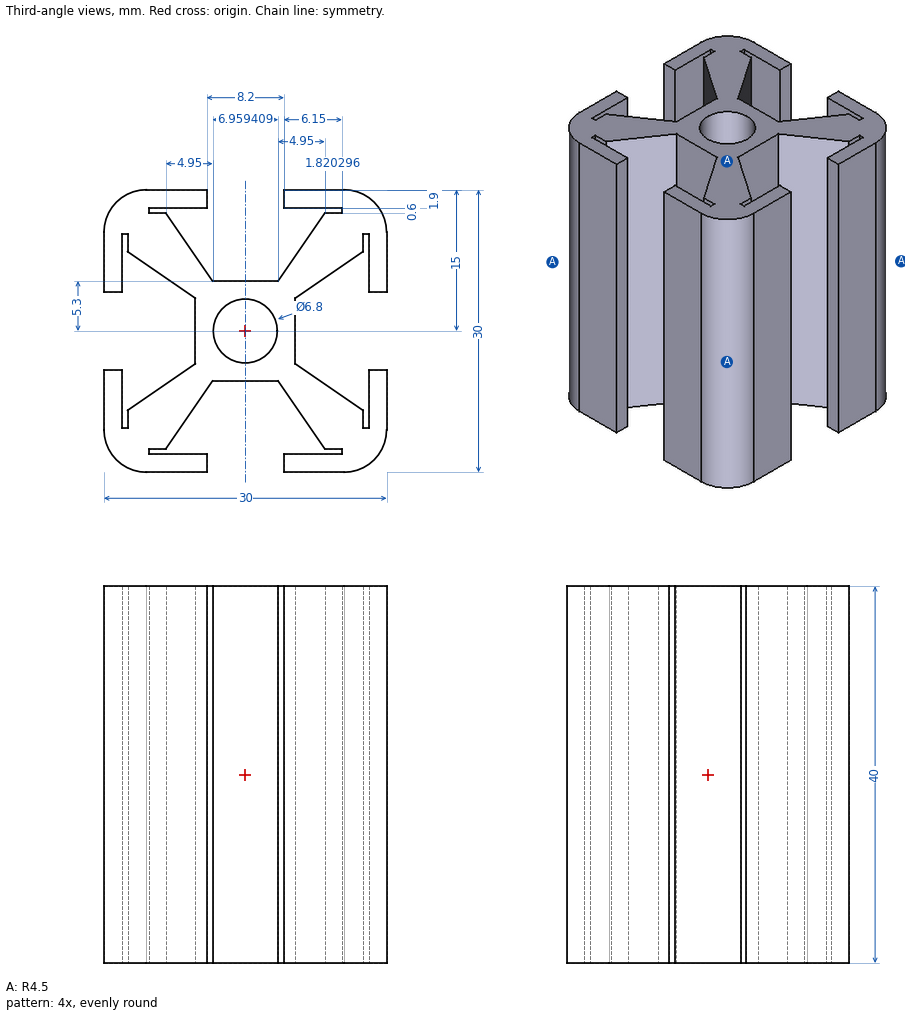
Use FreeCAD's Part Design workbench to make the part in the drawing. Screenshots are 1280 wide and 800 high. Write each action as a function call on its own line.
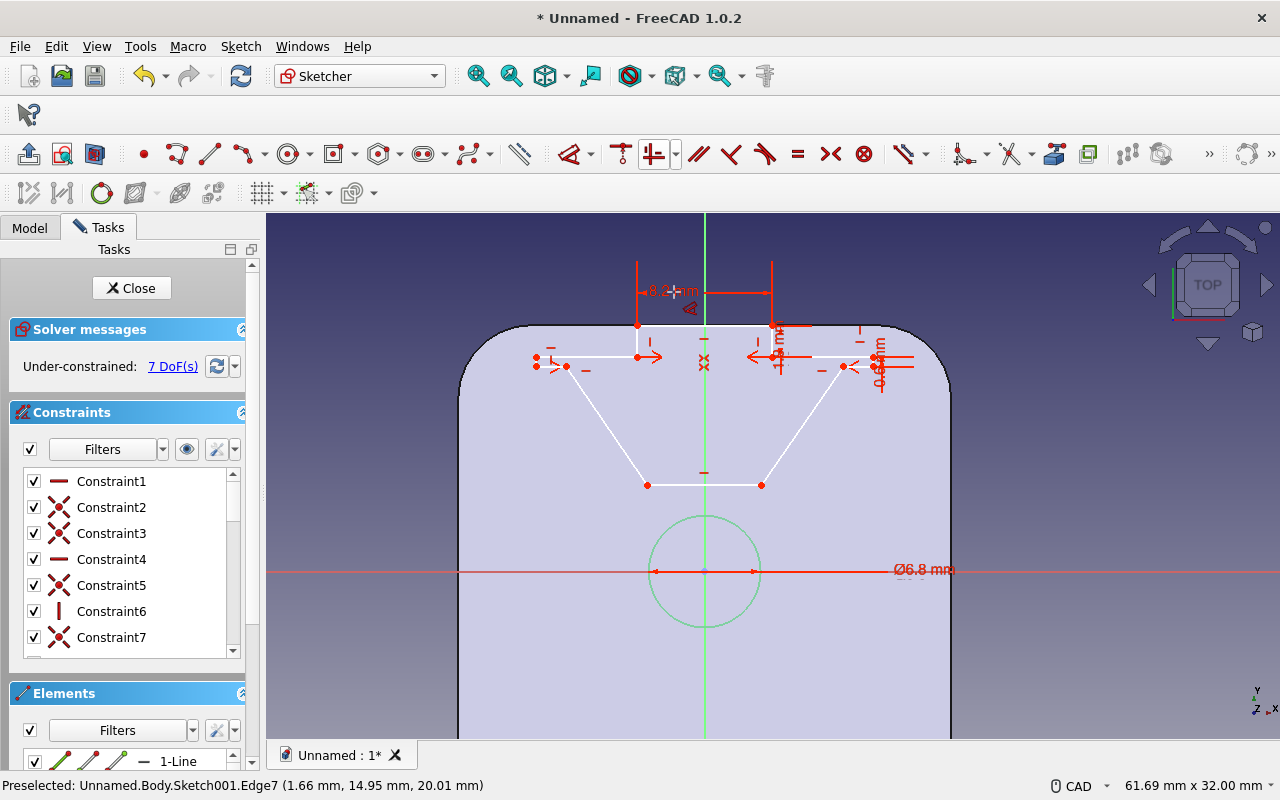
click(772, 326)
click(806, 449)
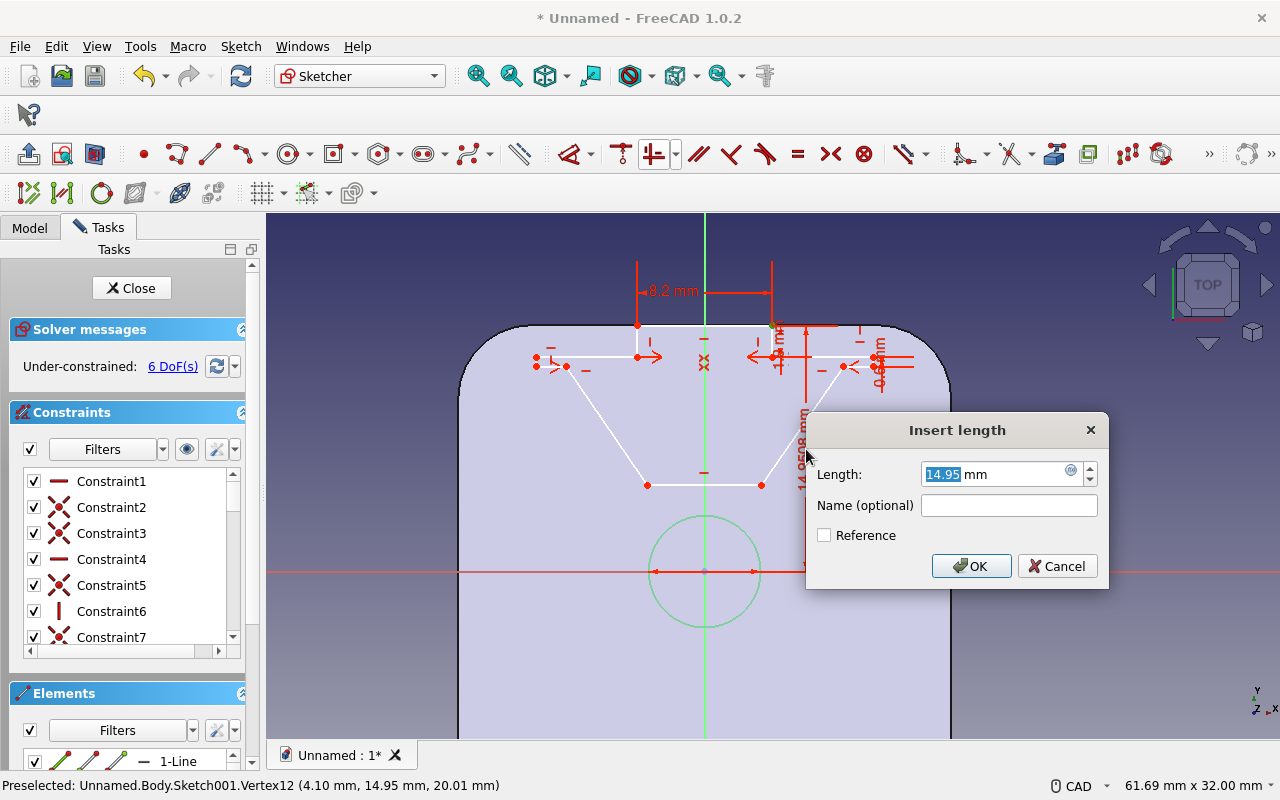
text(15)
key(Return)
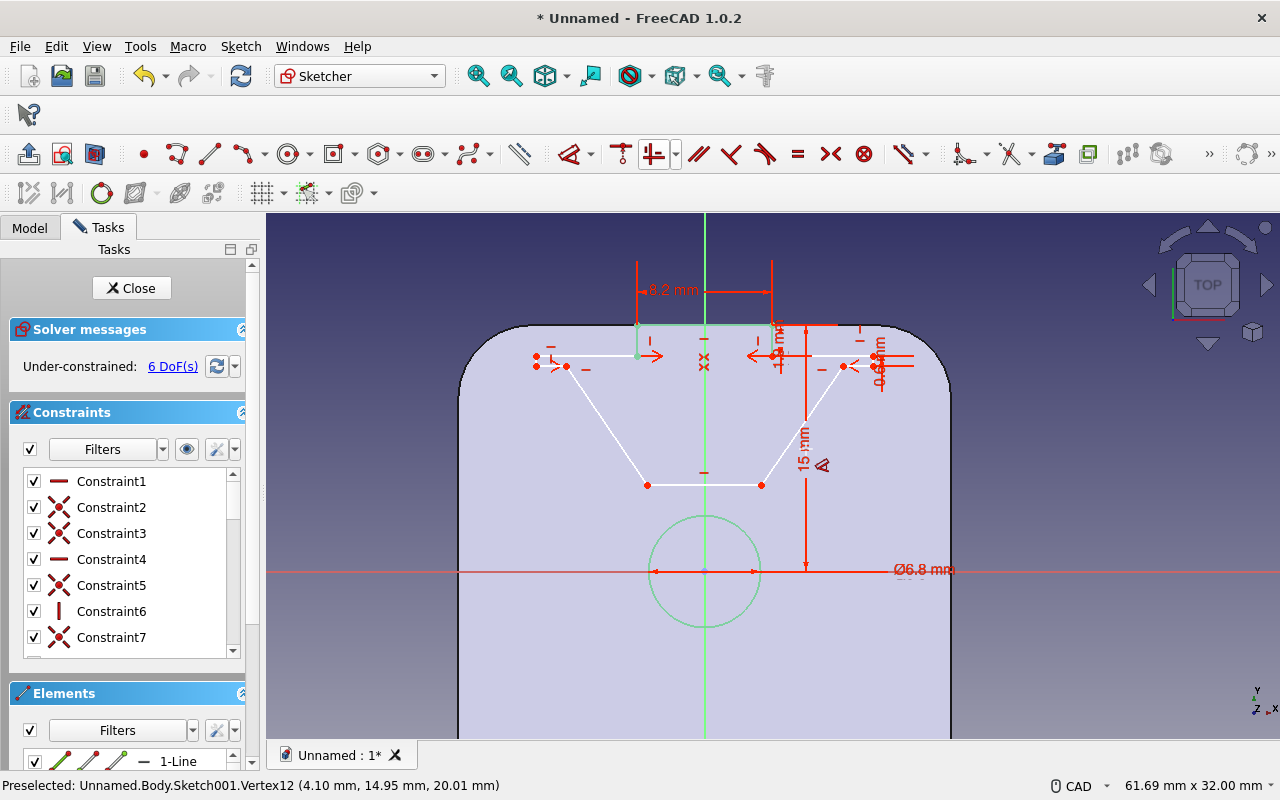
scroll(843, 356, up, 2)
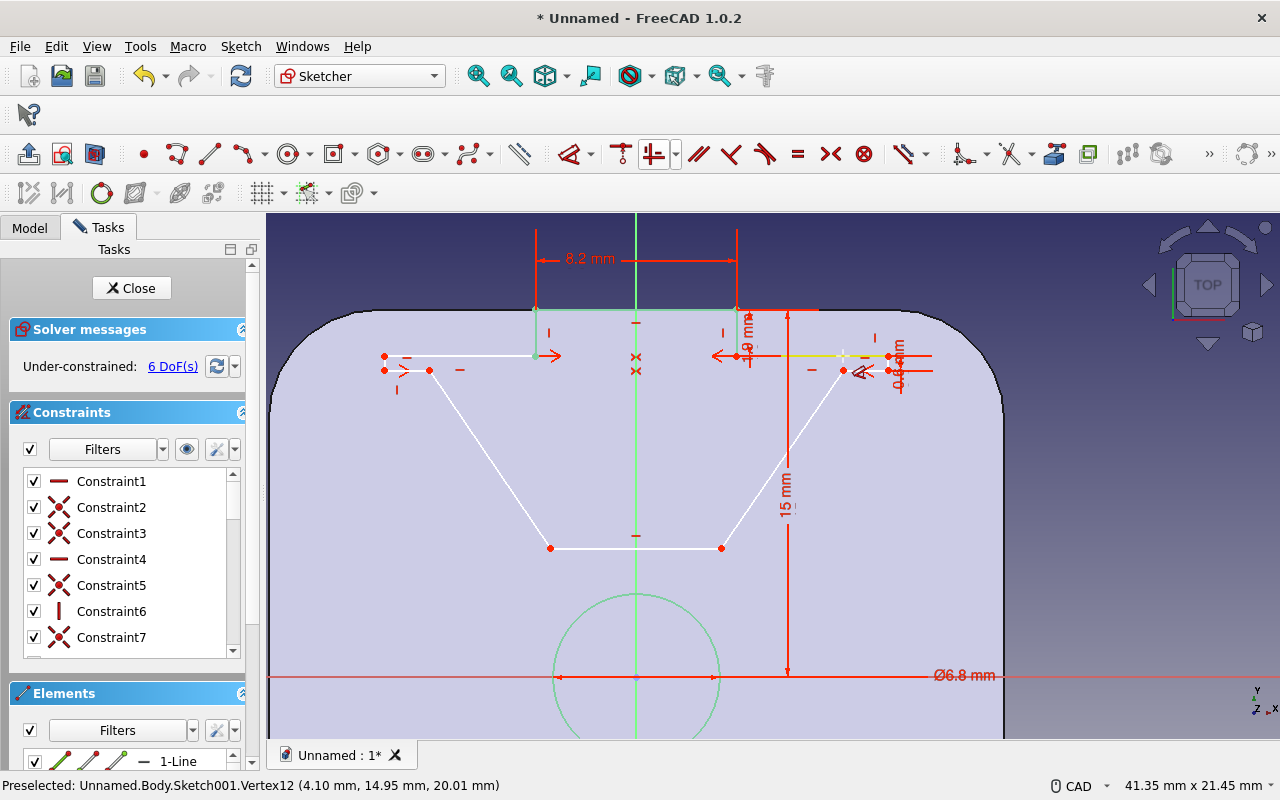
click(843, 356)
click(847, 322)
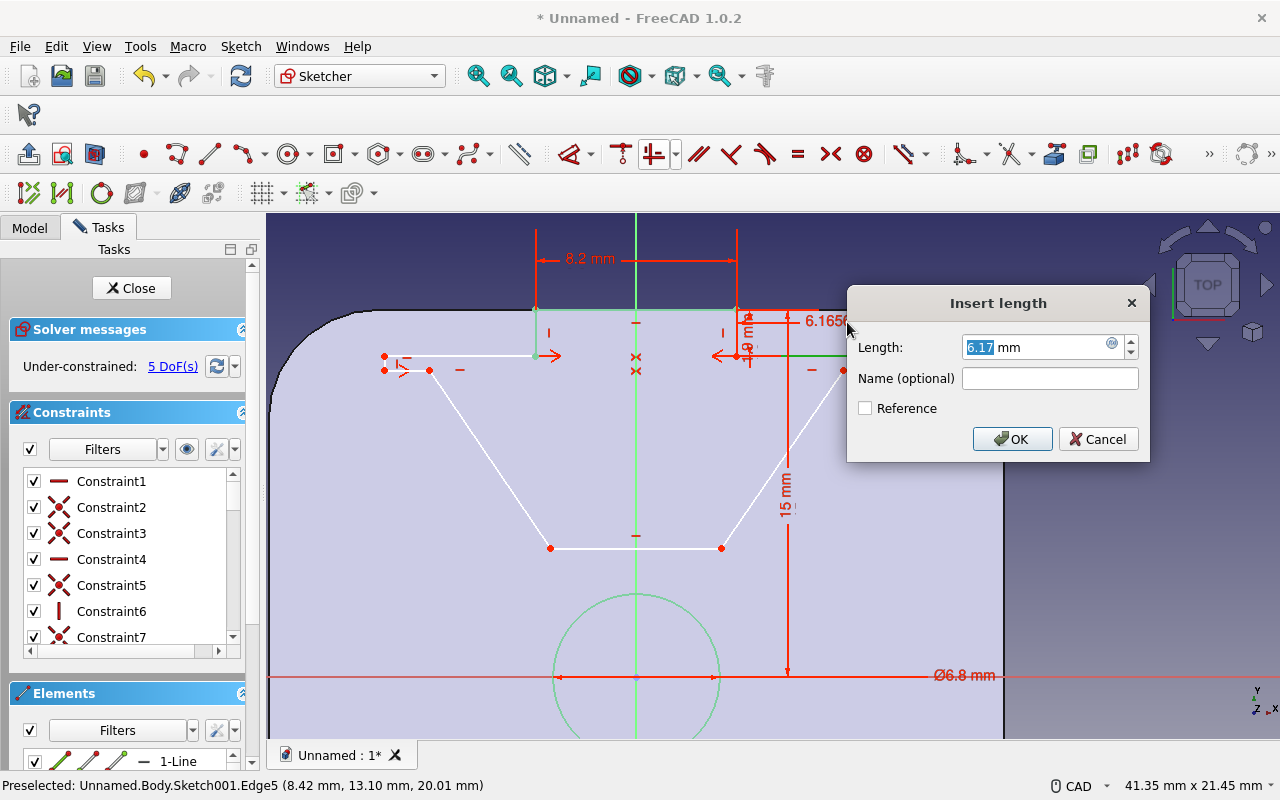
text(6.15)
key(Return)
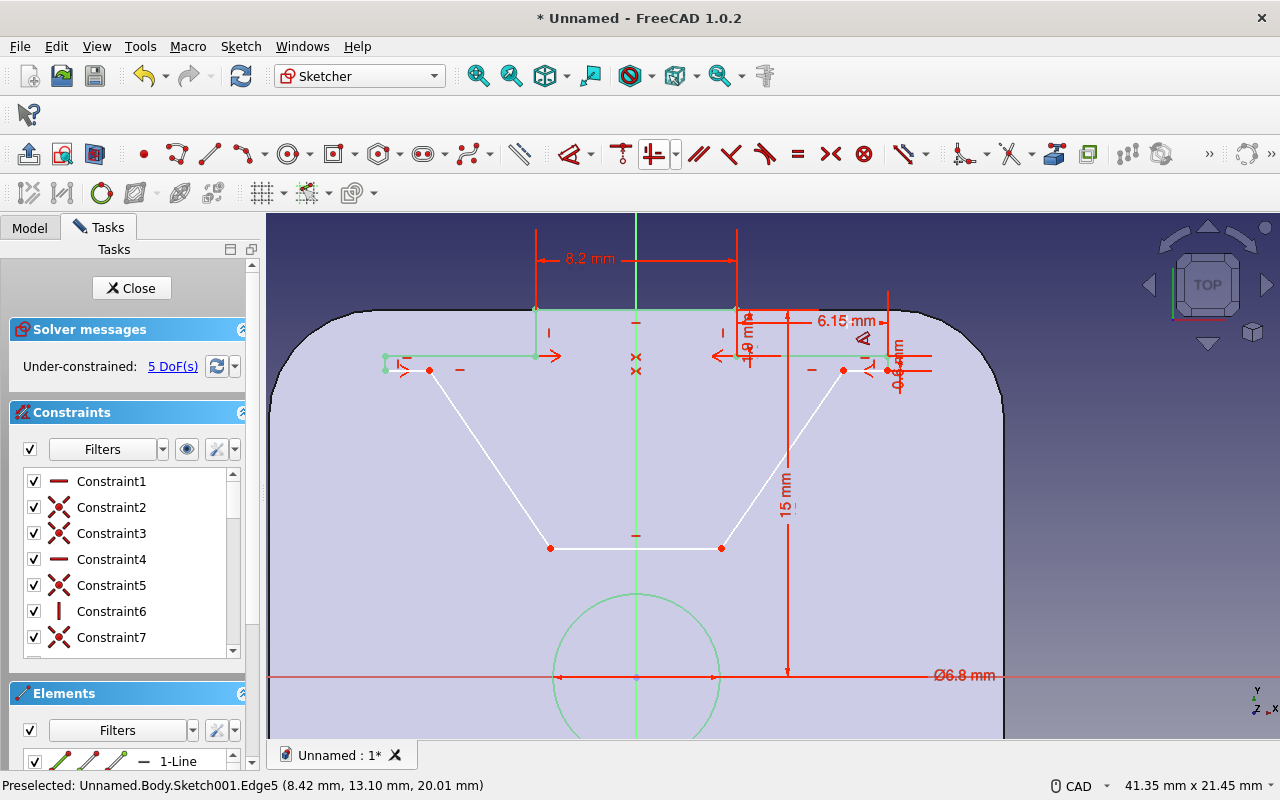
click(551, 549)
click(517, 613)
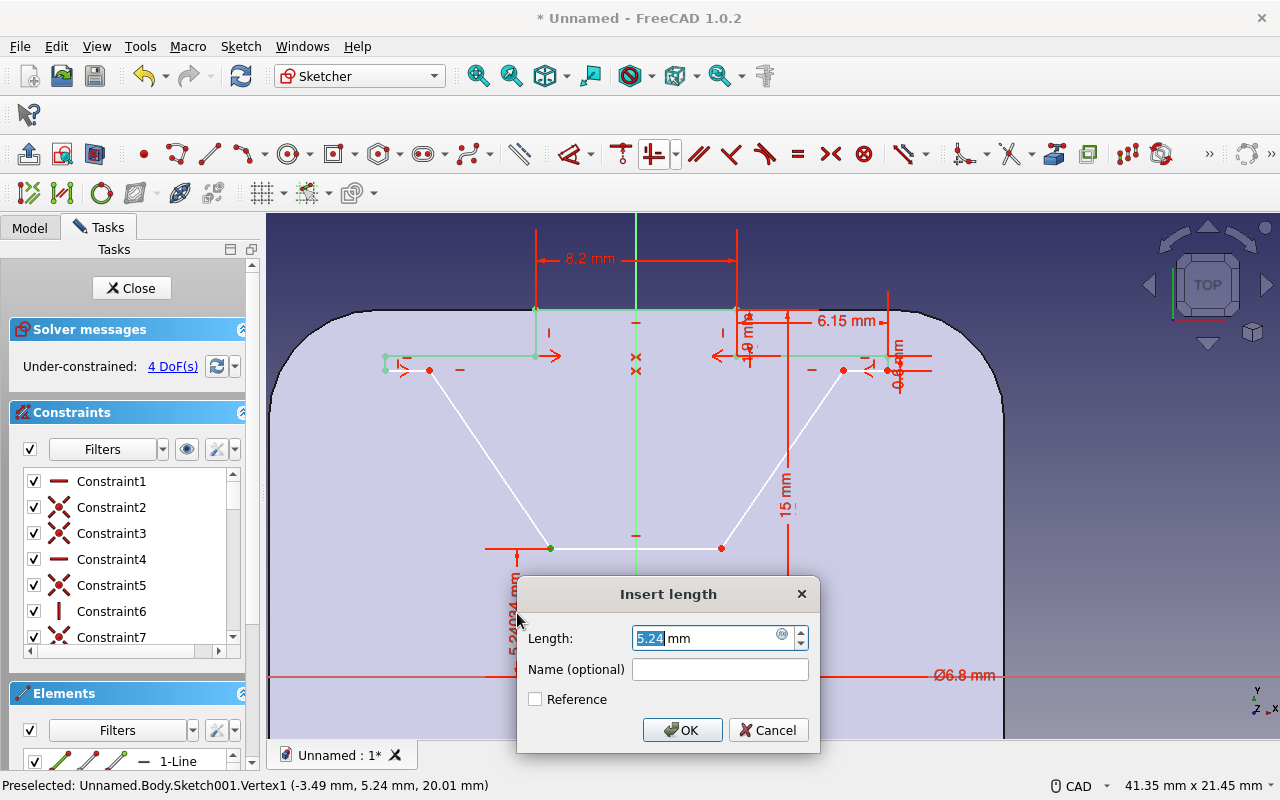
text(5.3)
key(Return)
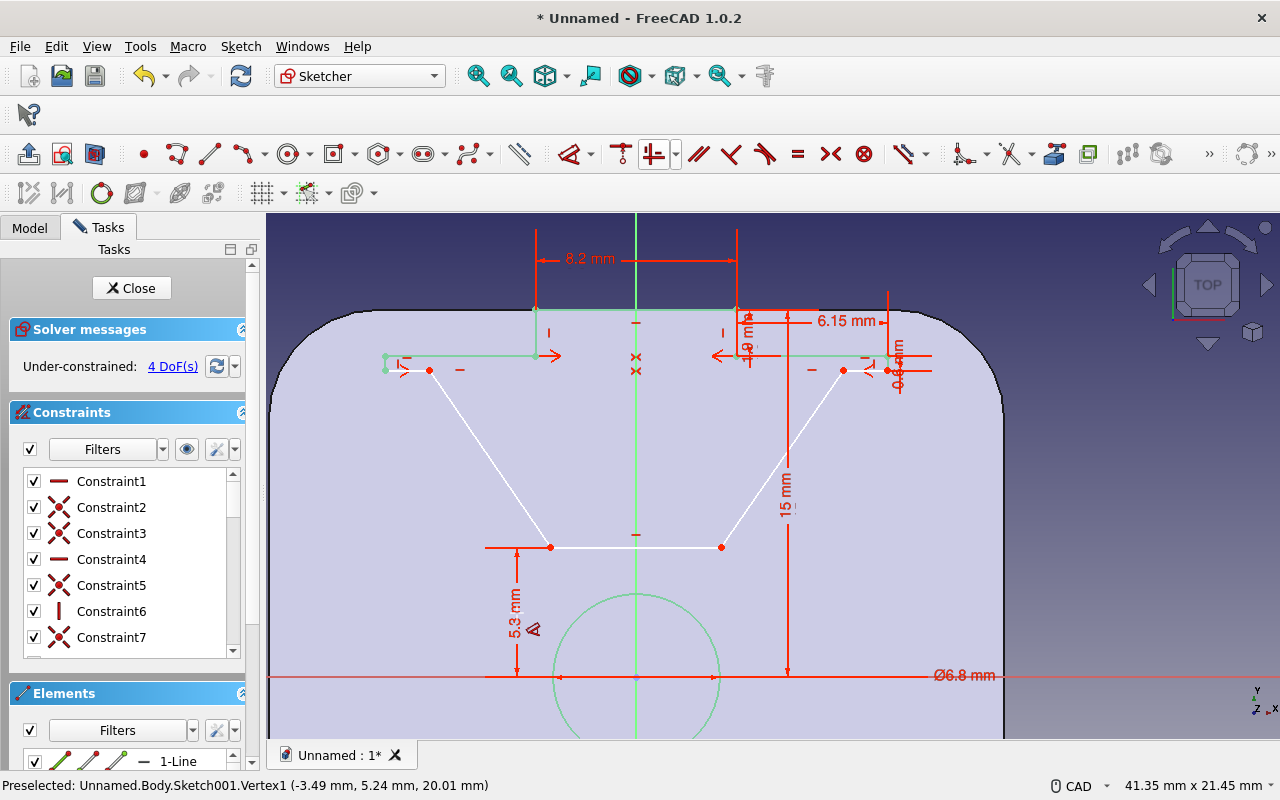
click(758, 495)
click(782, 582)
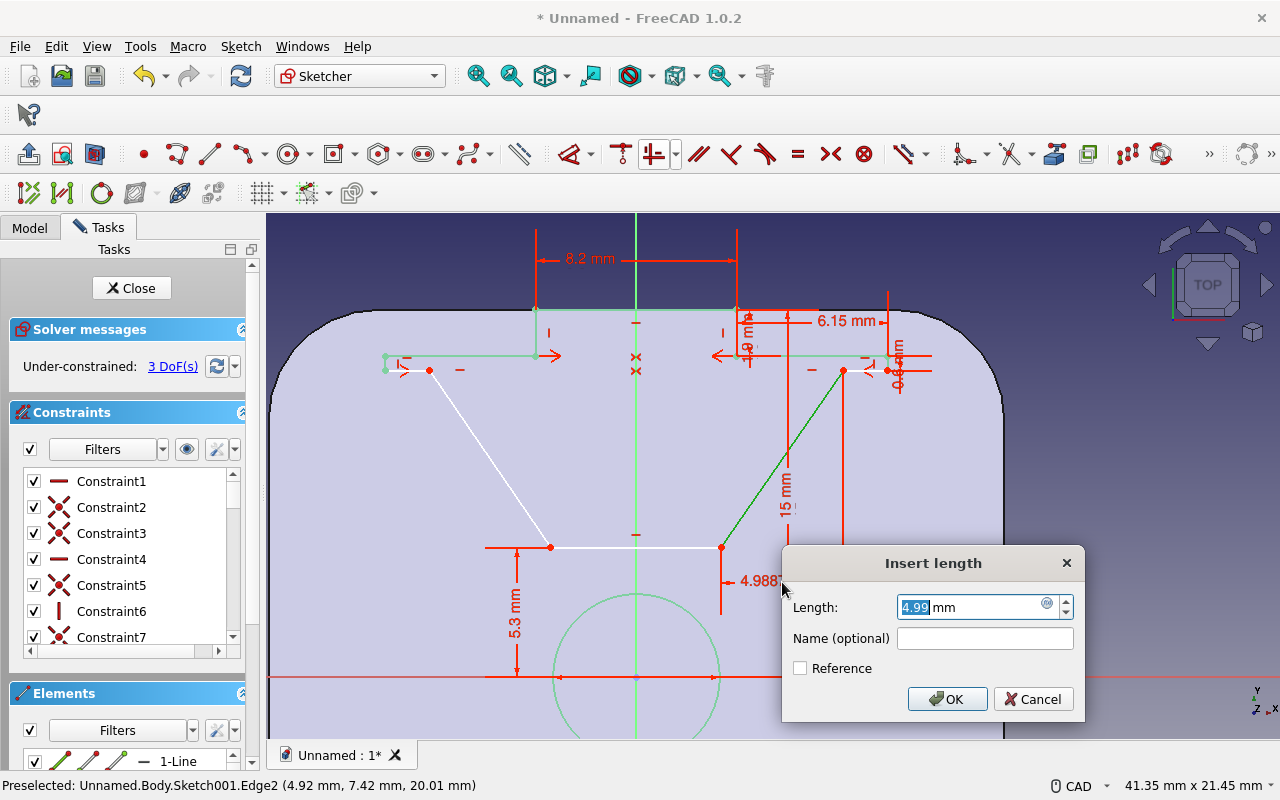
text(4.95)
key(Return)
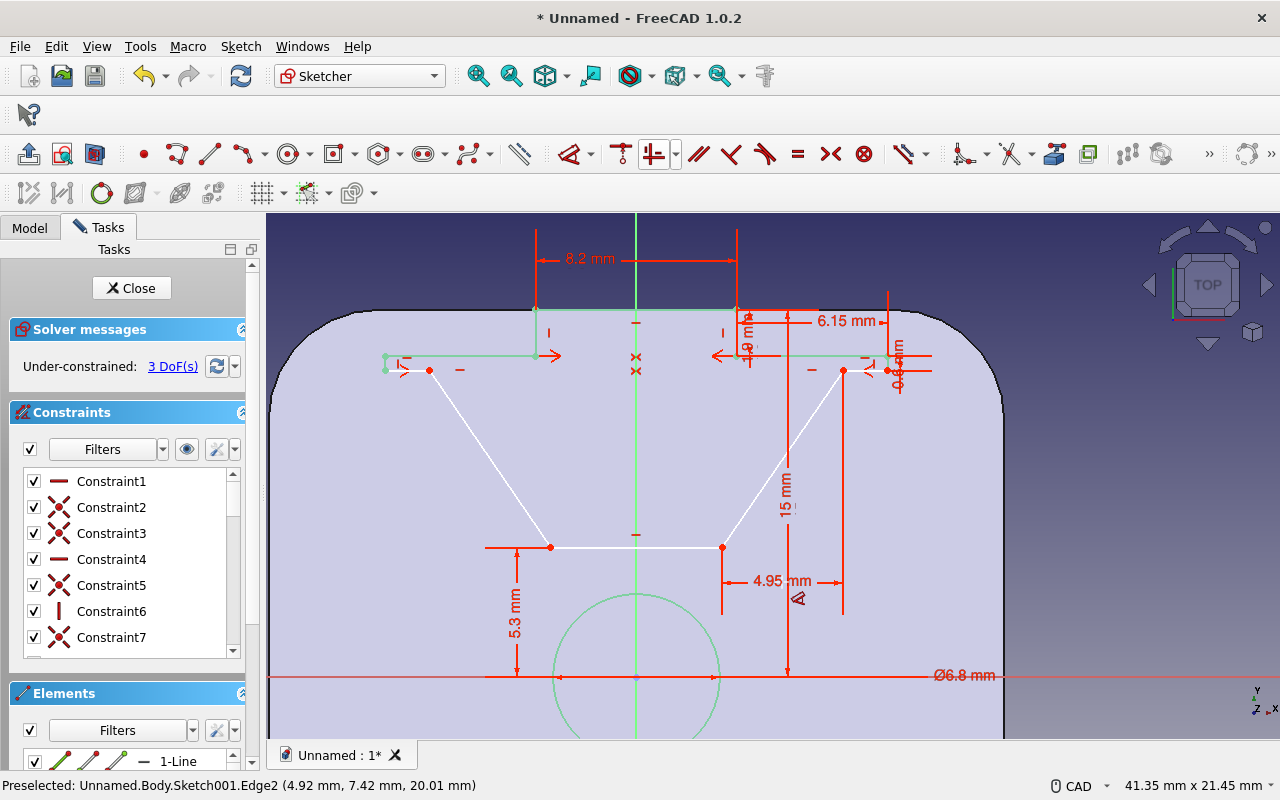
click(466, 424)
click(490, 337)